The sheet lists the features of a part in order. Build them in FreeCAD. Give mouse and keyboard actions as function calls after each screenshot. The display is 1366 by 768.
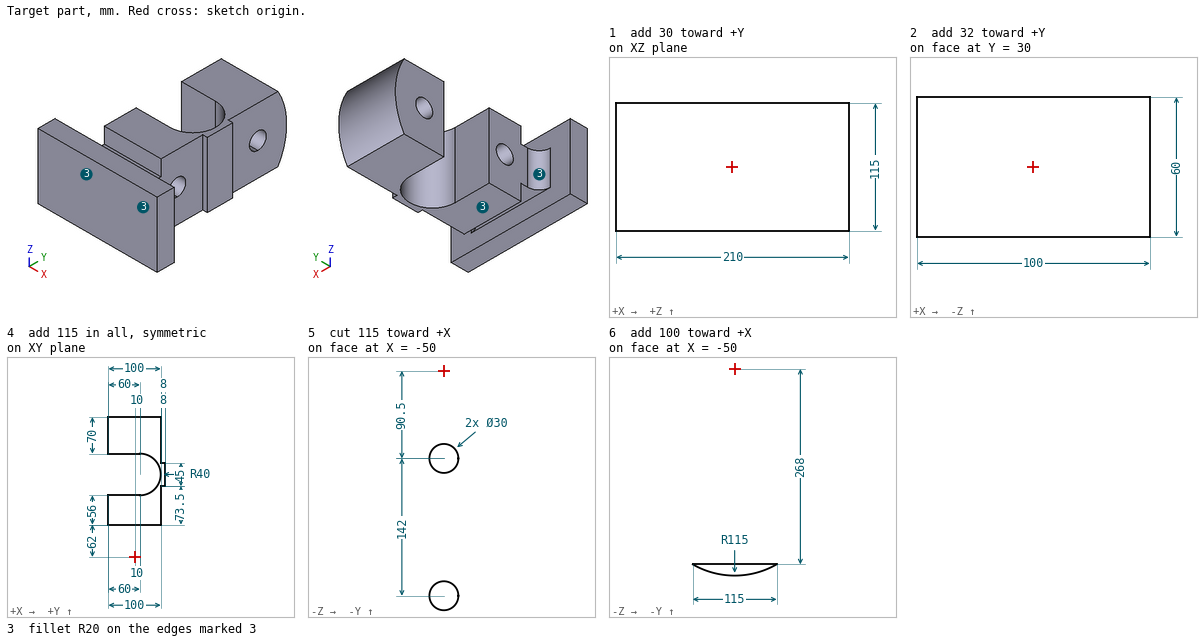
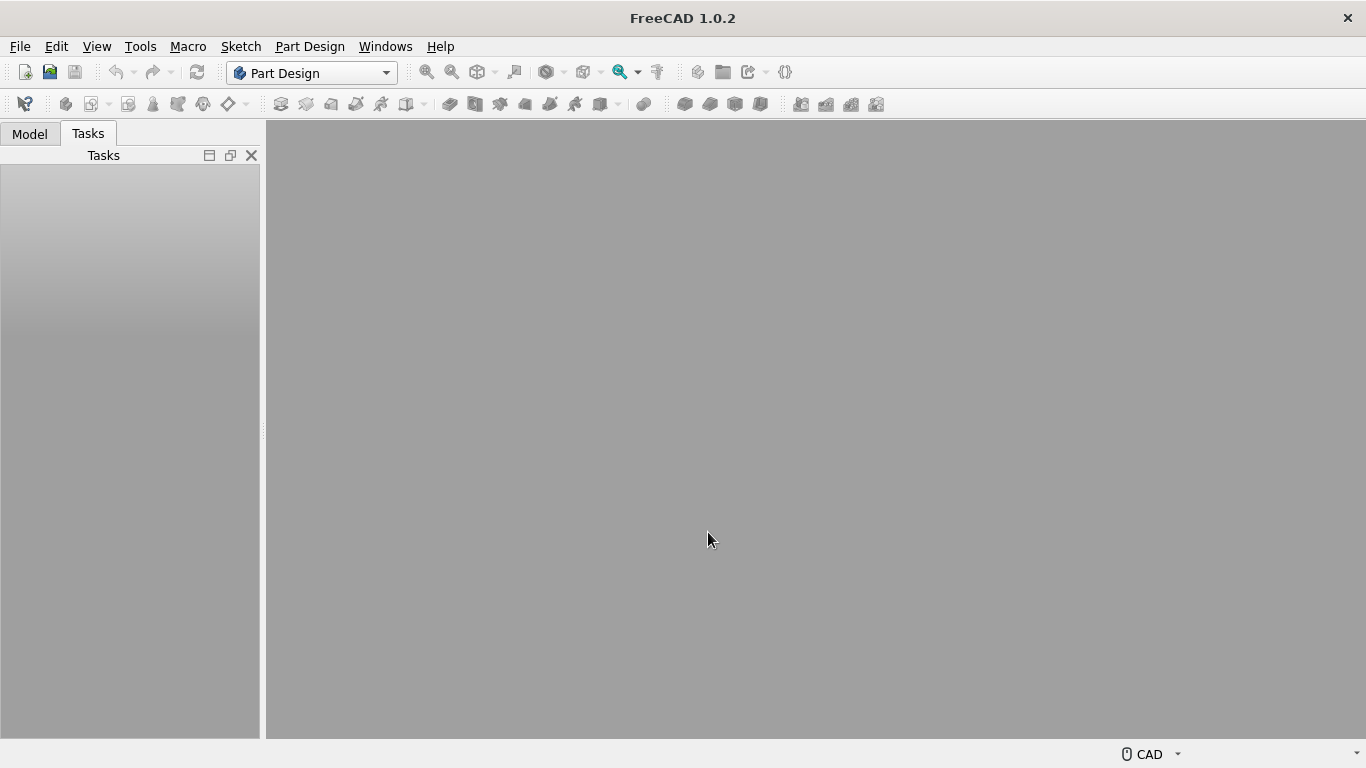
key(ctrl+n)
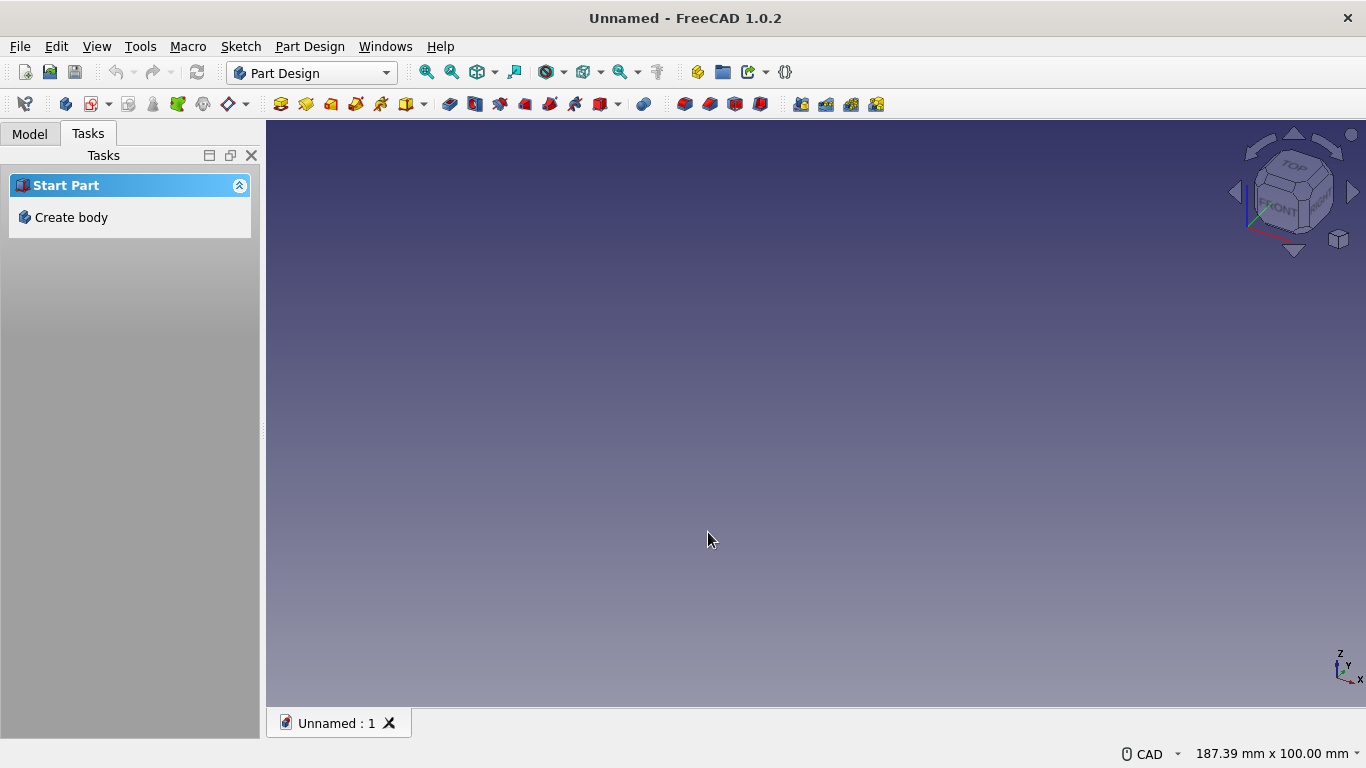
click(90, 104)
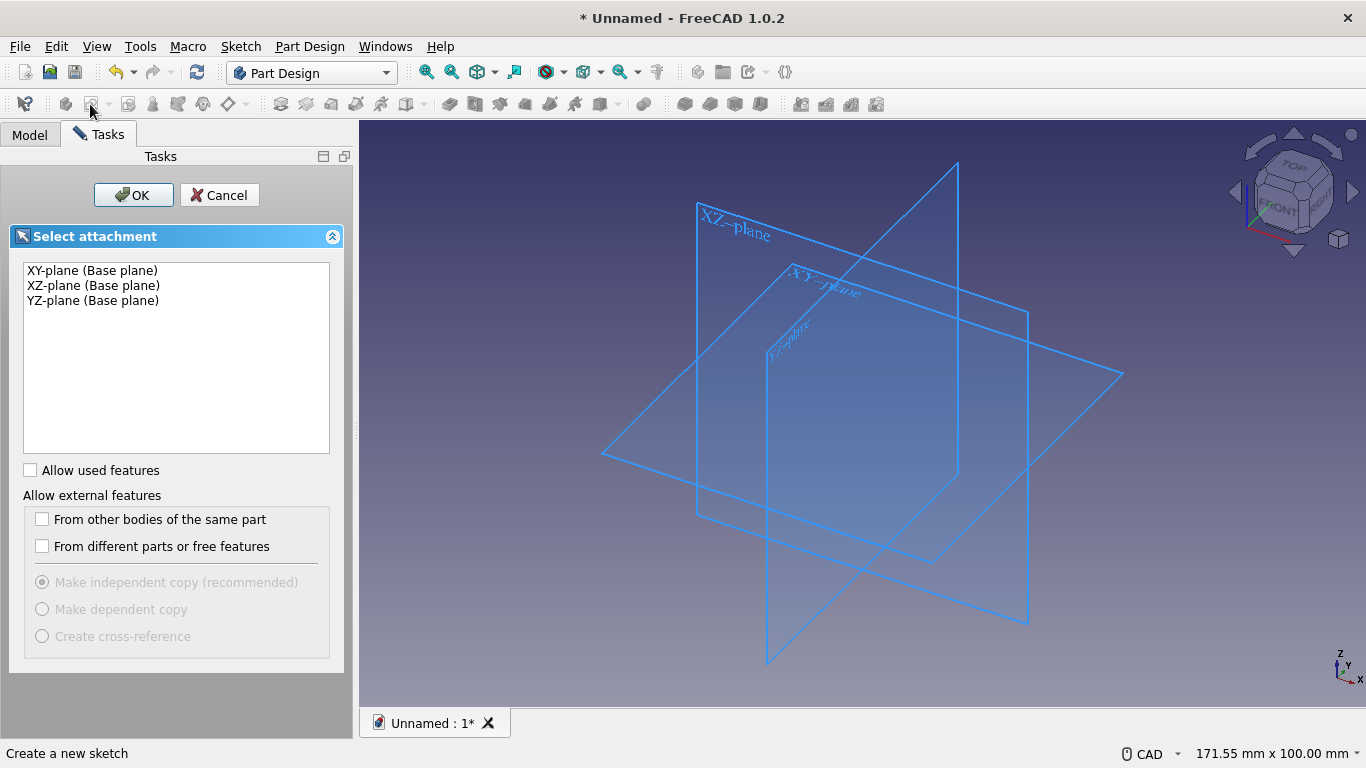
click(84, 286)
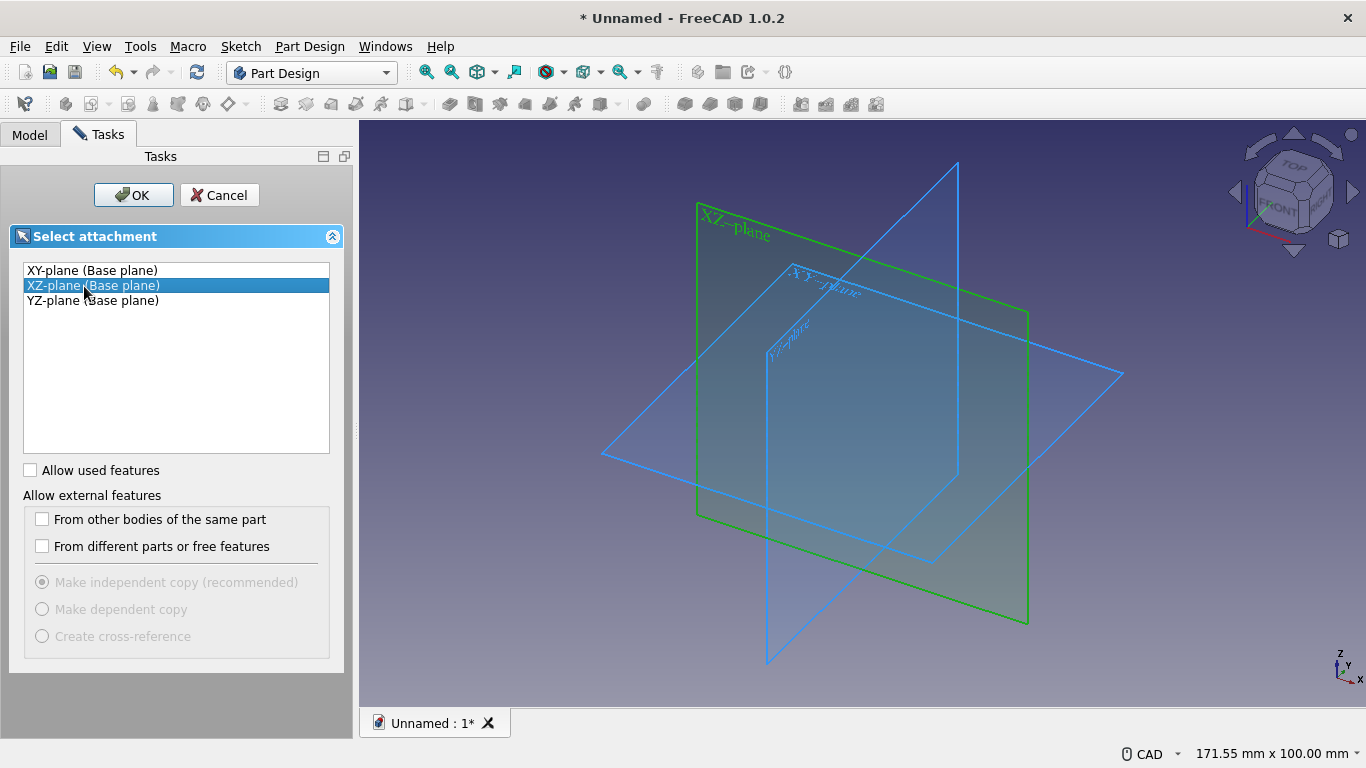
click(134, 195)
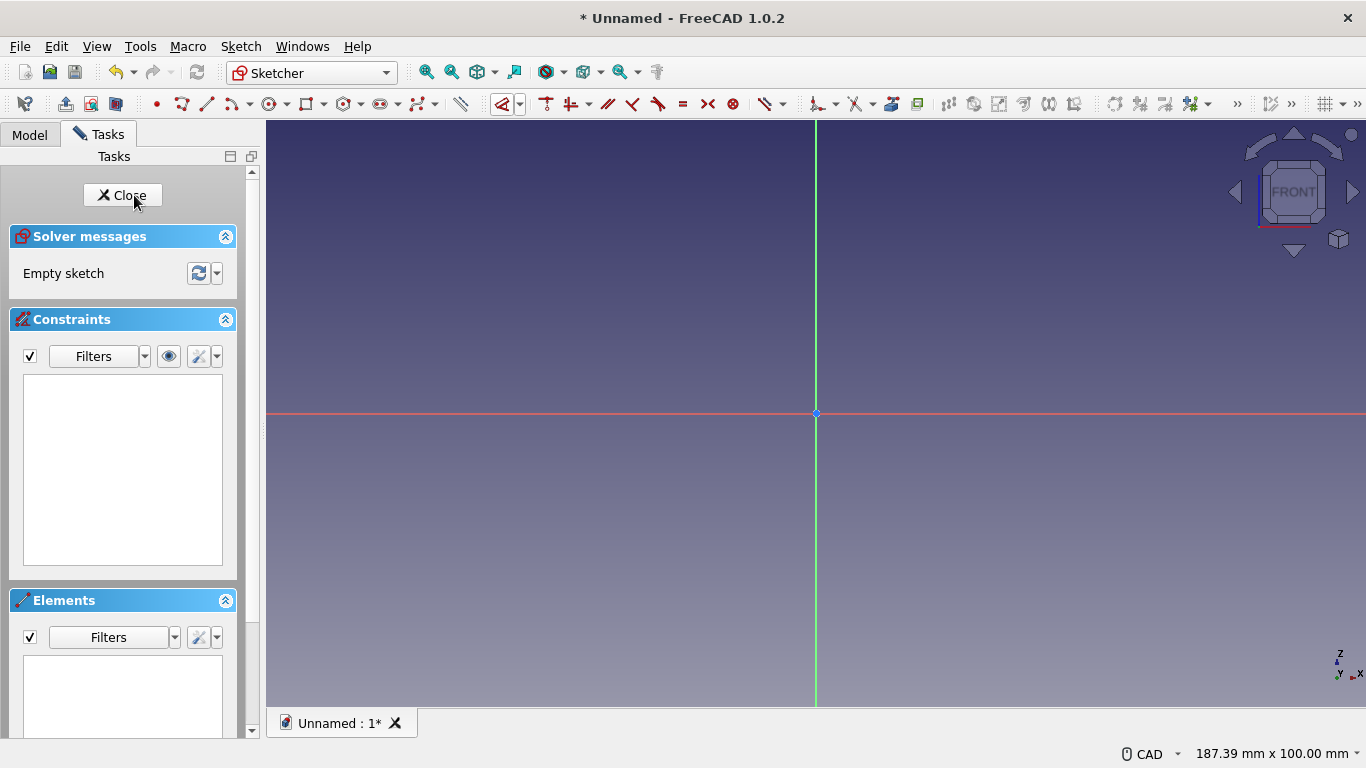
scroll(664, 414, down, 3)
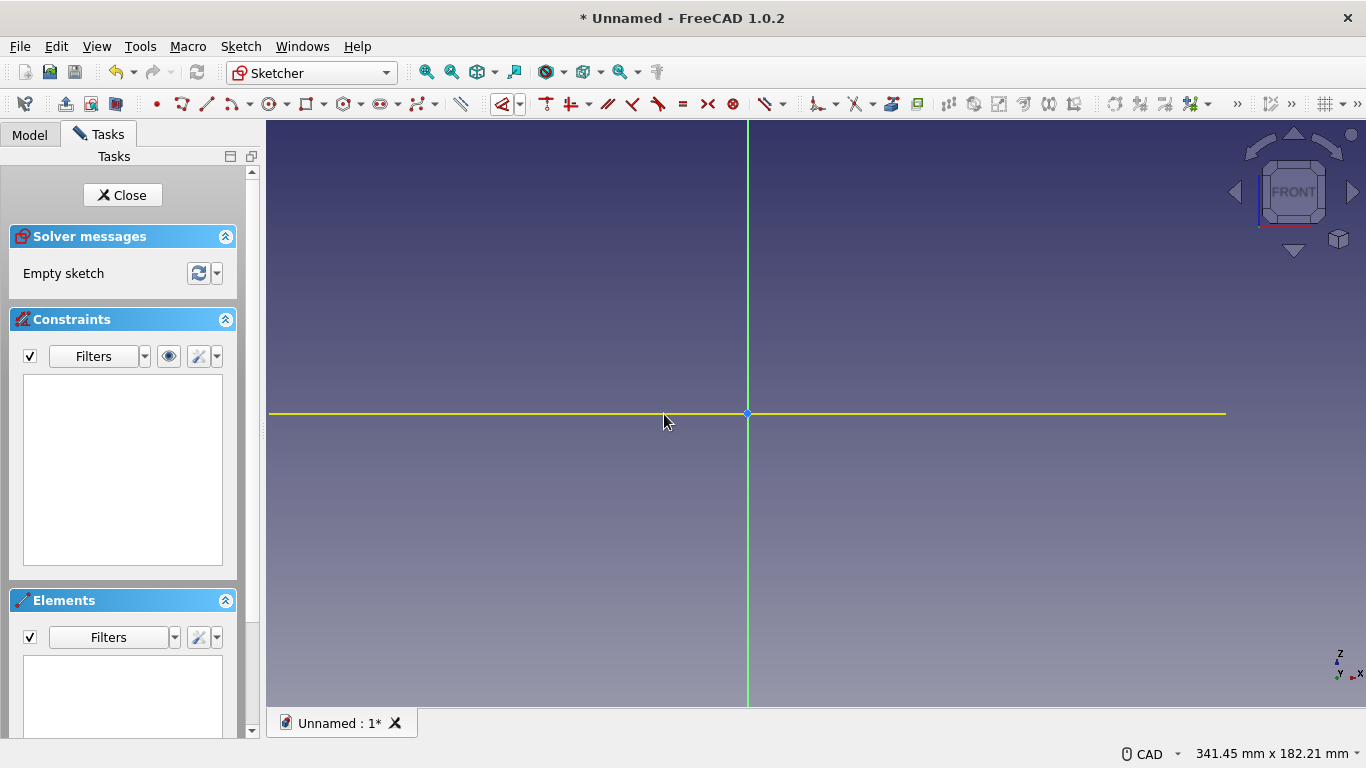
key(g)
key(v)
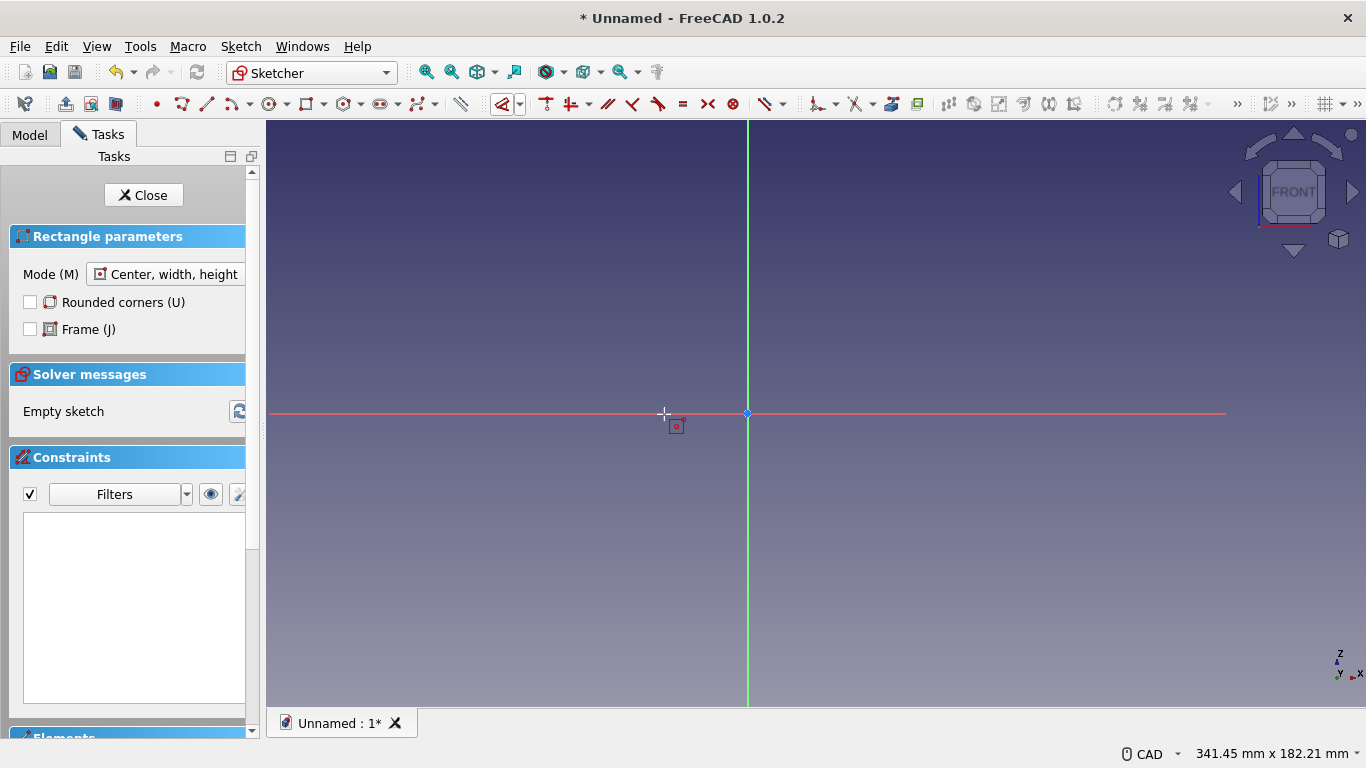
click(748, 414)
move(1086, 229)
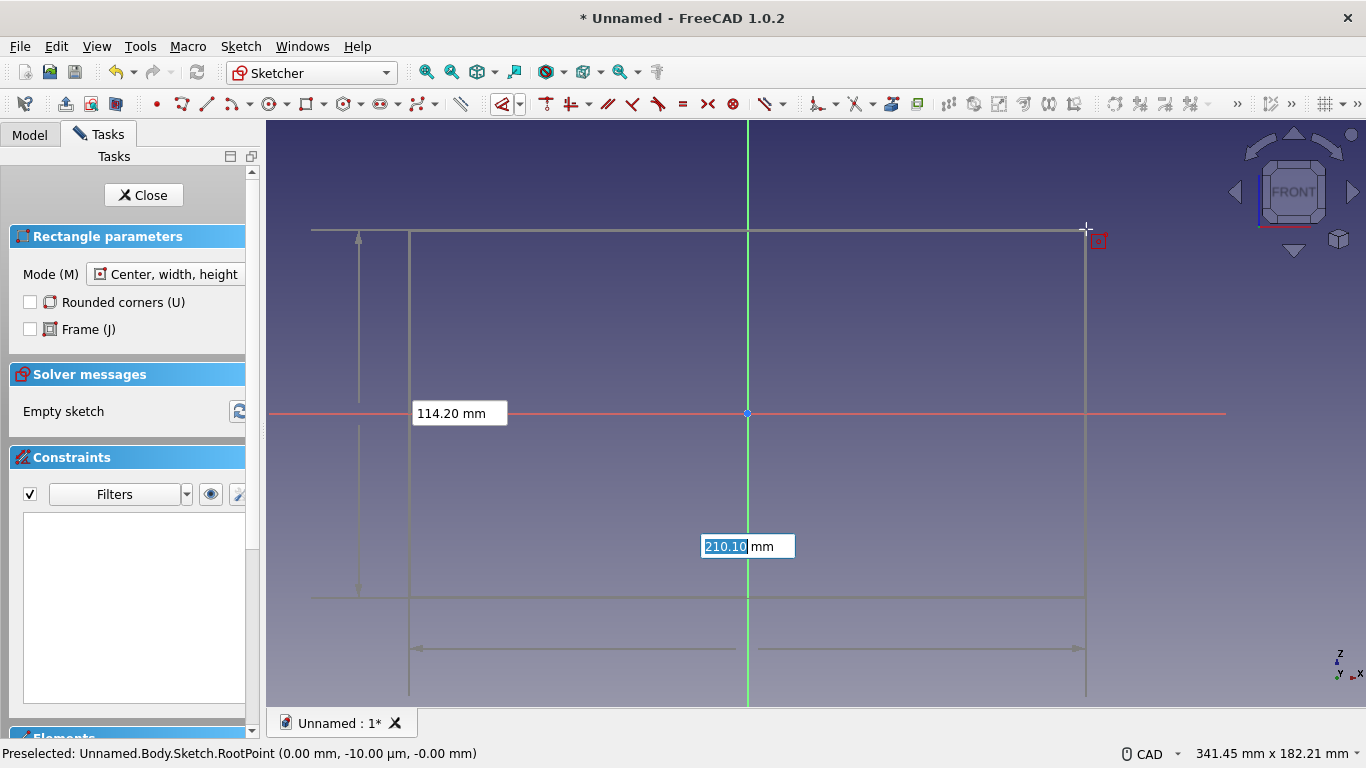
text(210)
key(Tab)
text(115)
key(Return)
key(Escape)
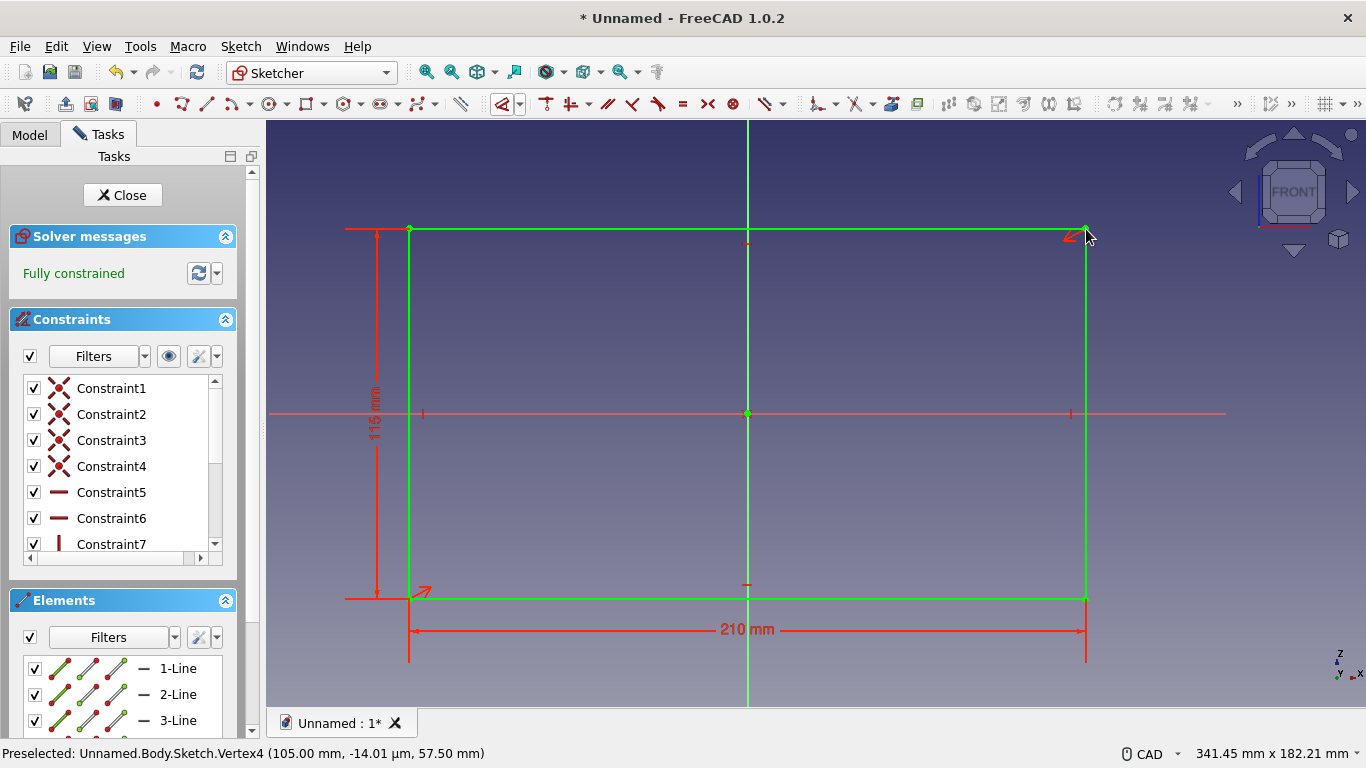
click(123, 195)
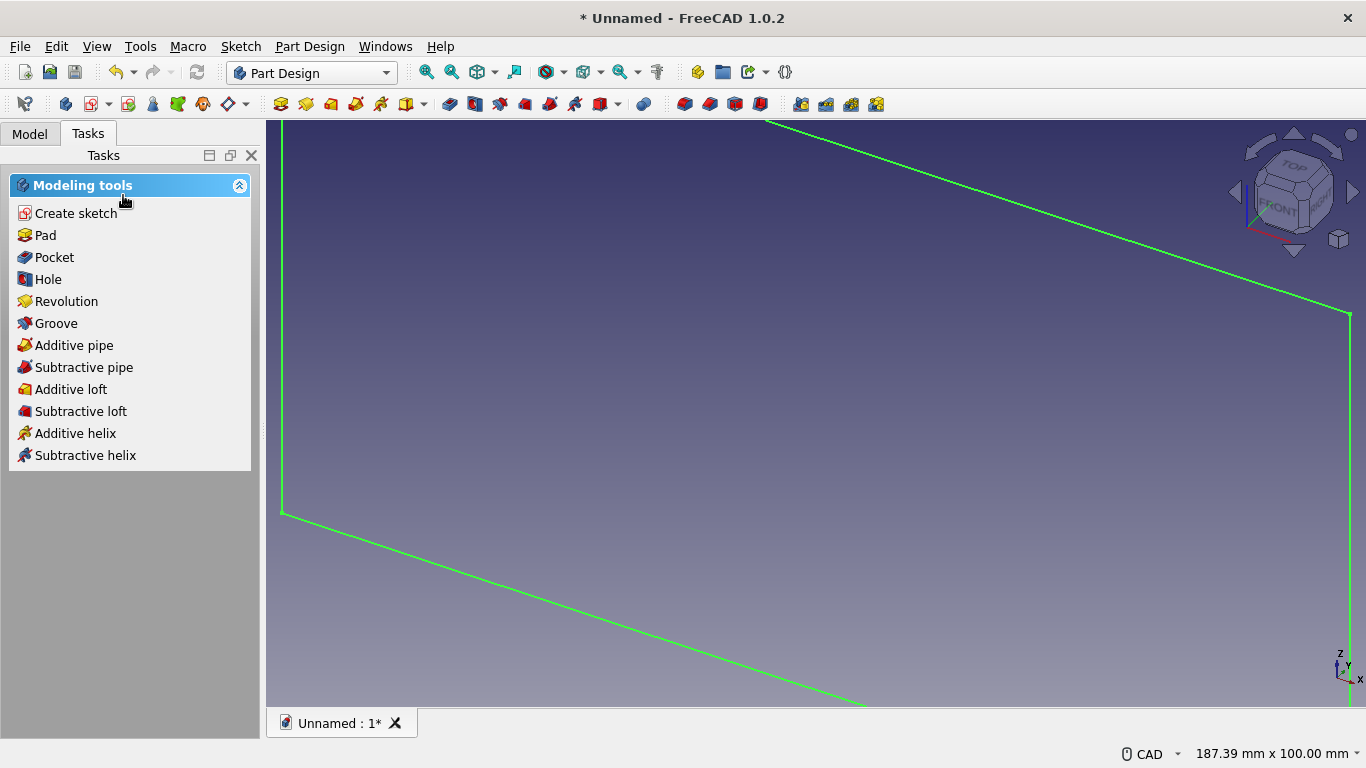
click(281, 104)